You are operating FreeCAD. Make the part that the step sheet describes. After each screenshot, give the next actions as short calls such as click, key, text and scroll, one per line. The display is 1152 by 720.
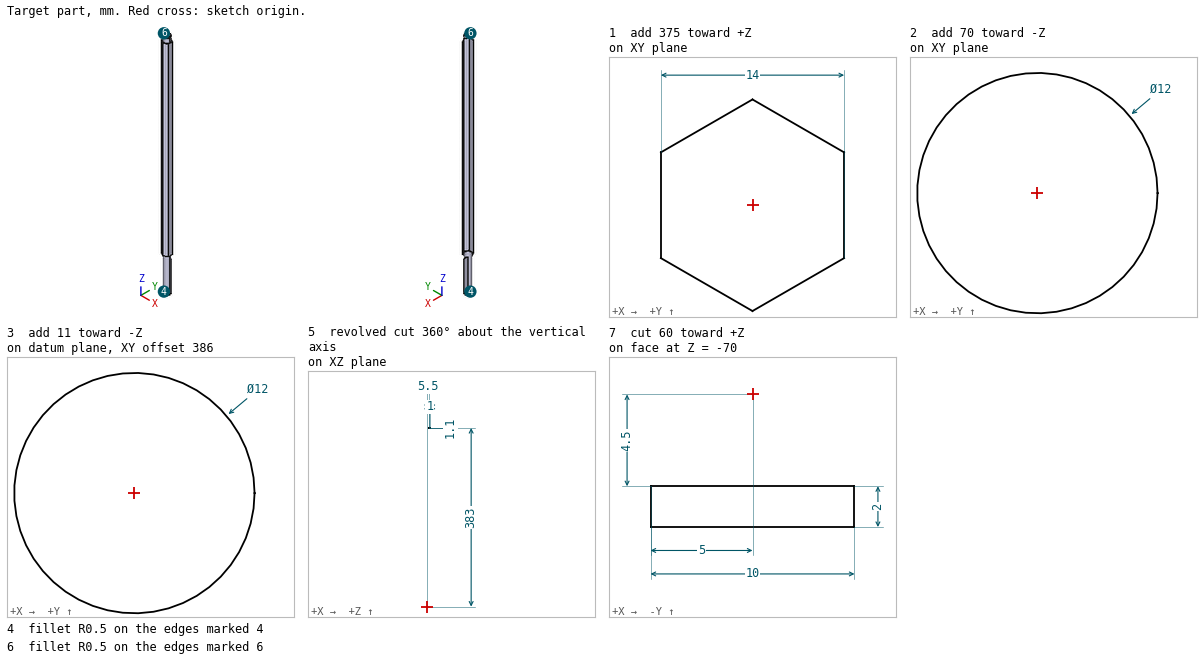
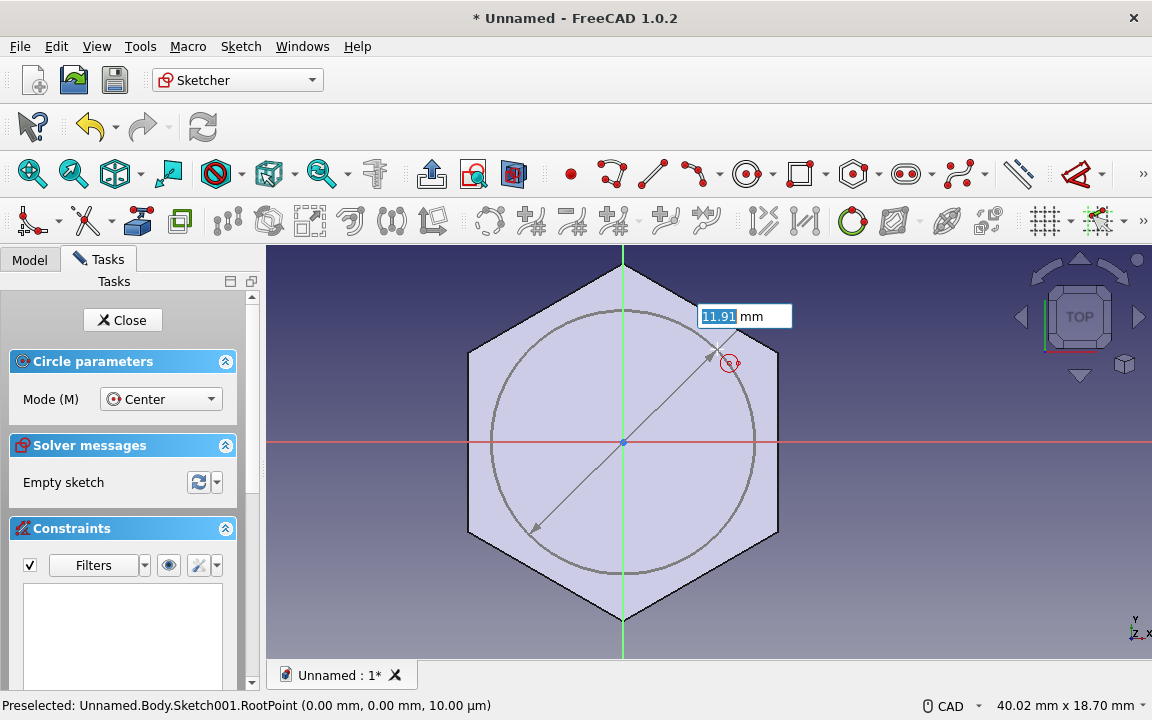
text(12)
key(Return)
key(Escape)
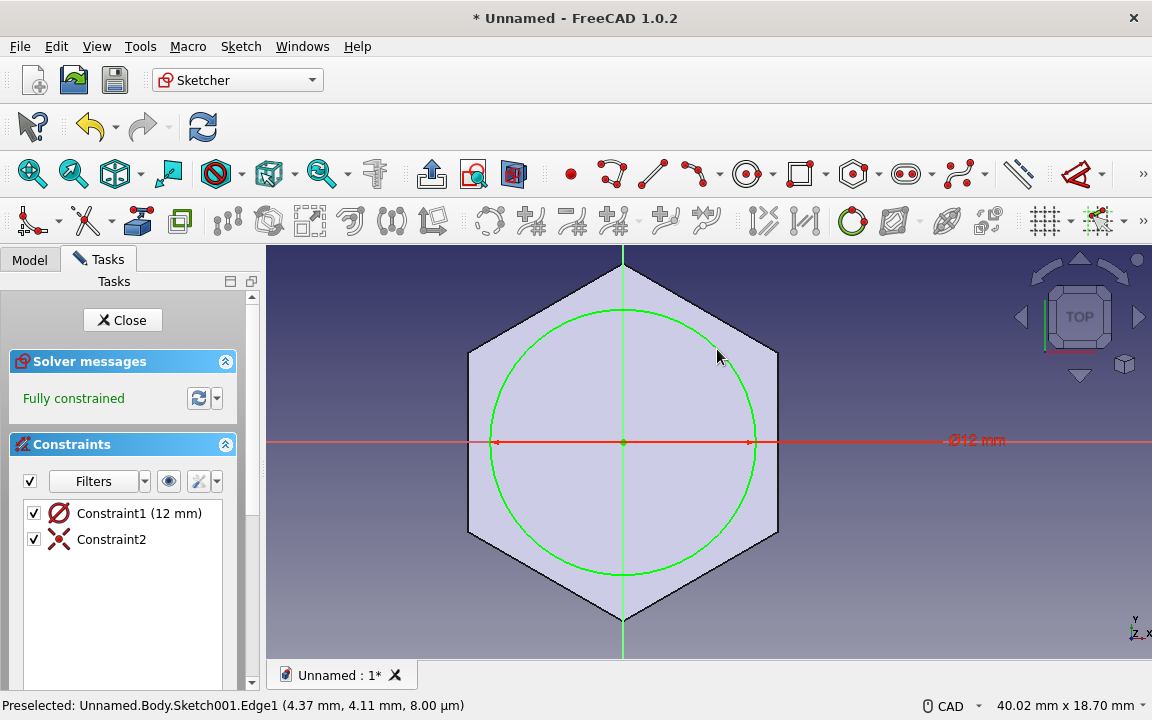
click(123, 320)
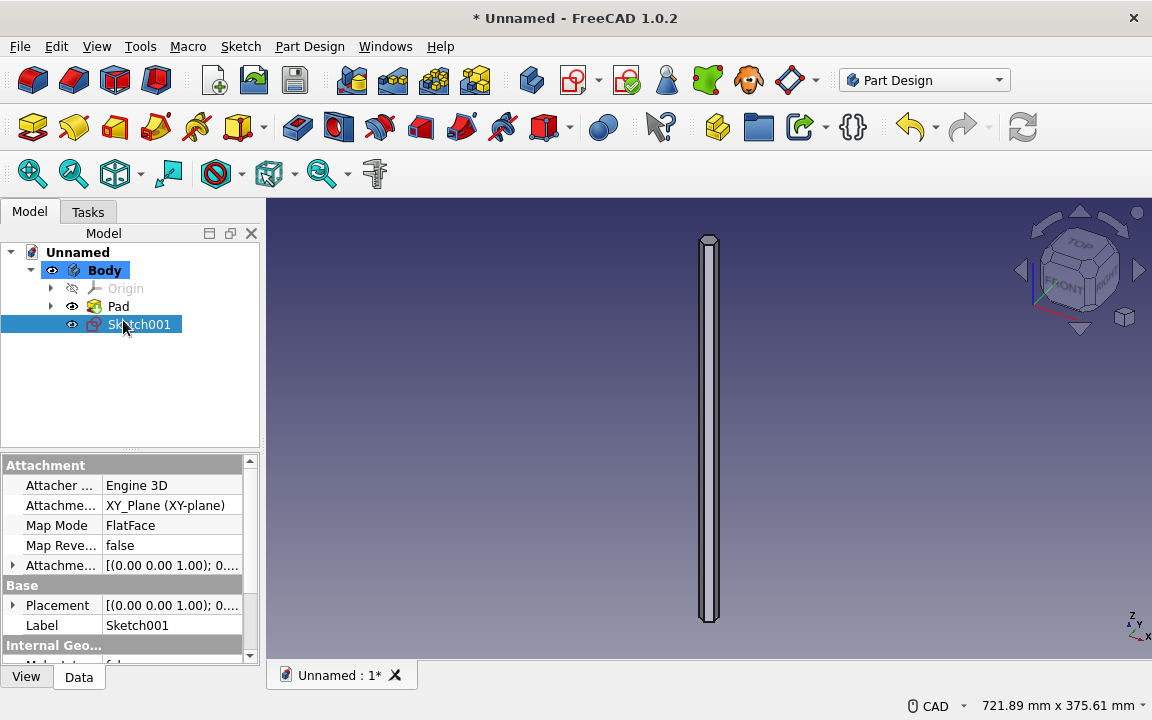
click(33, 128)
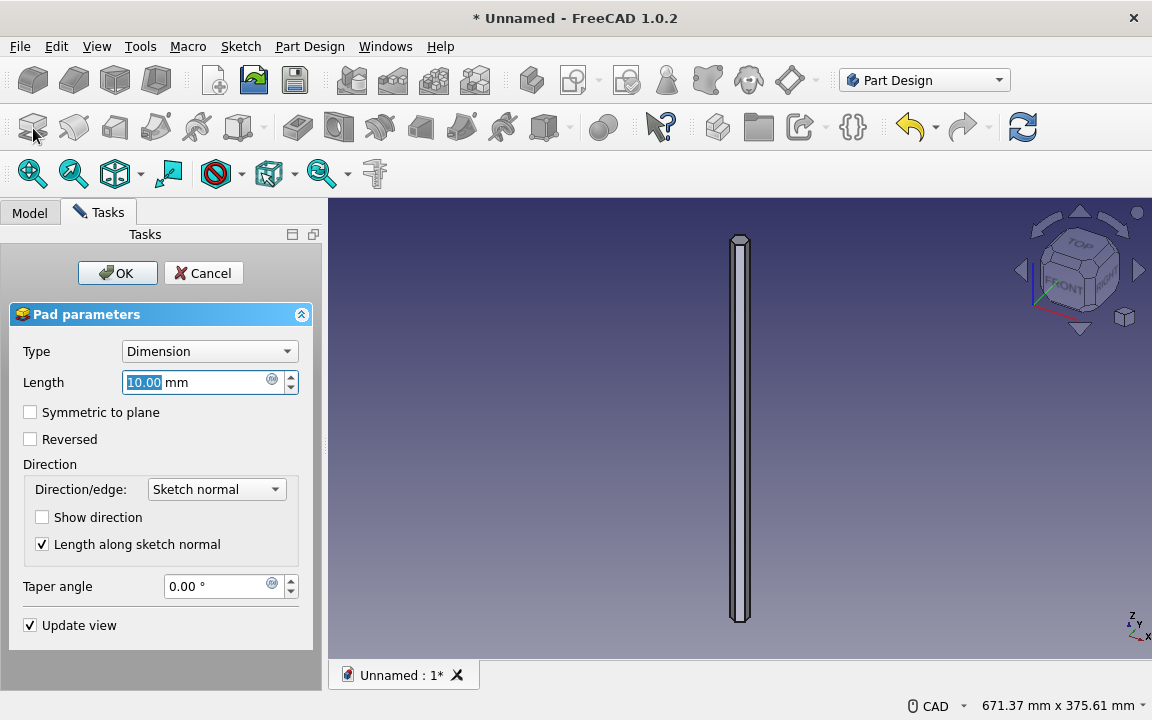
text(70)
key(Tab)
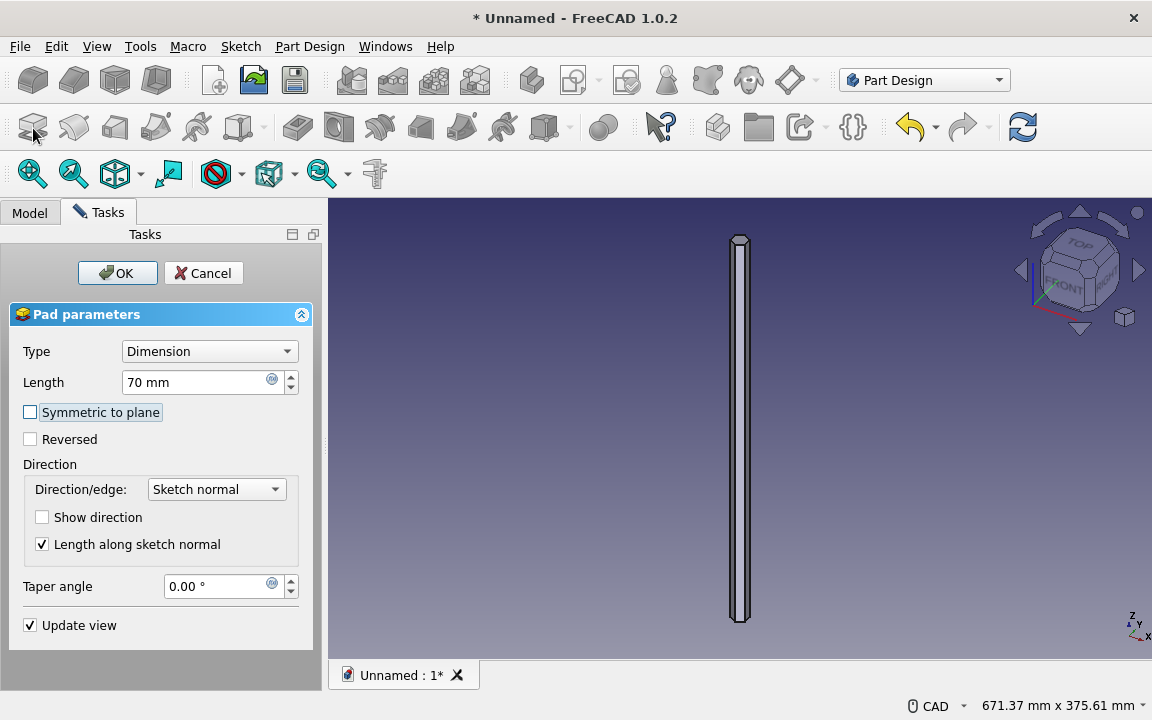
click(31, 439)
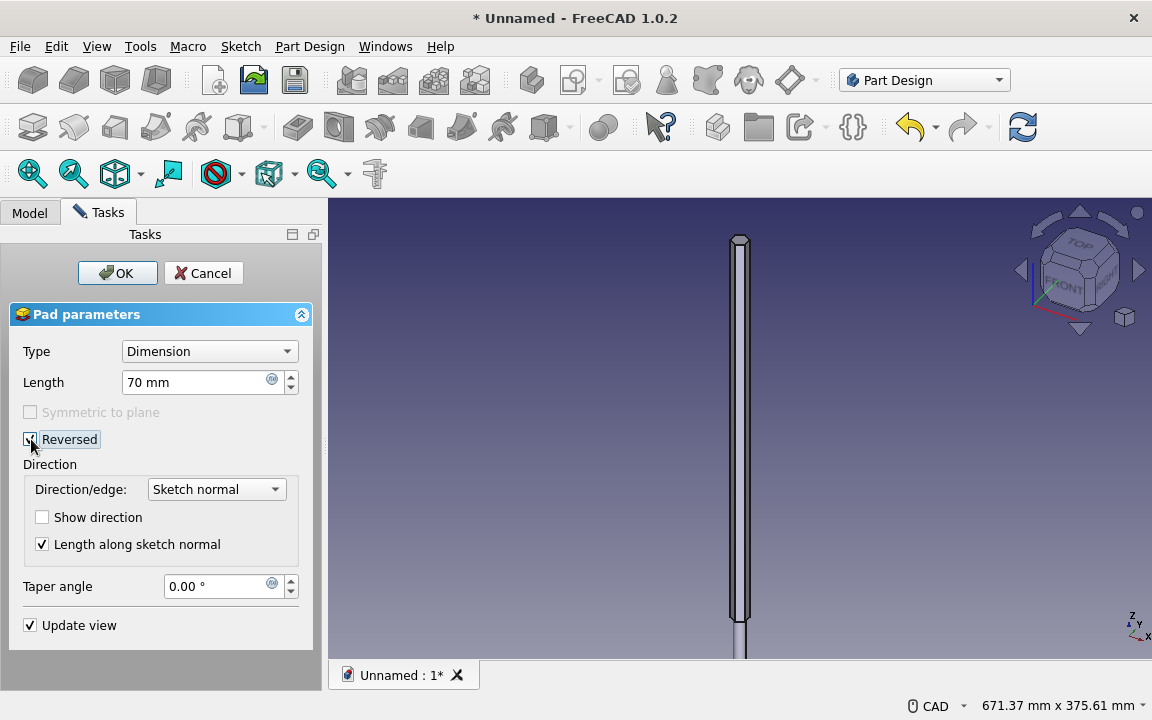
click(118, 273)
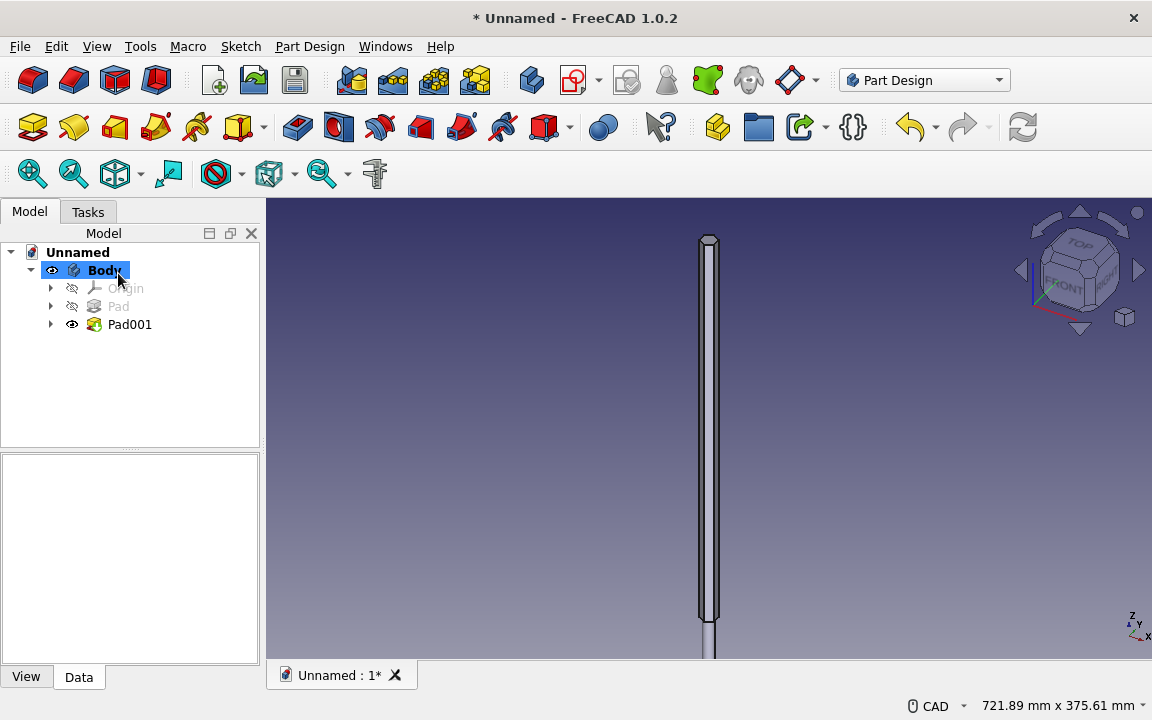
click(33, 174)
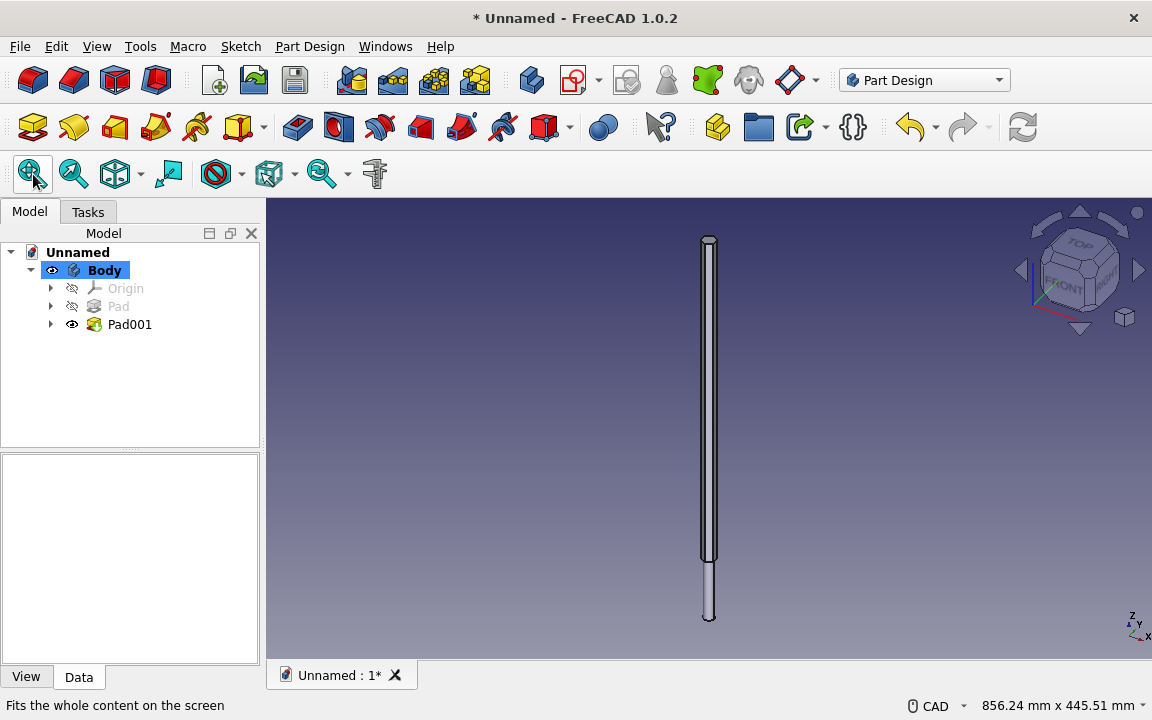
click(51, 288)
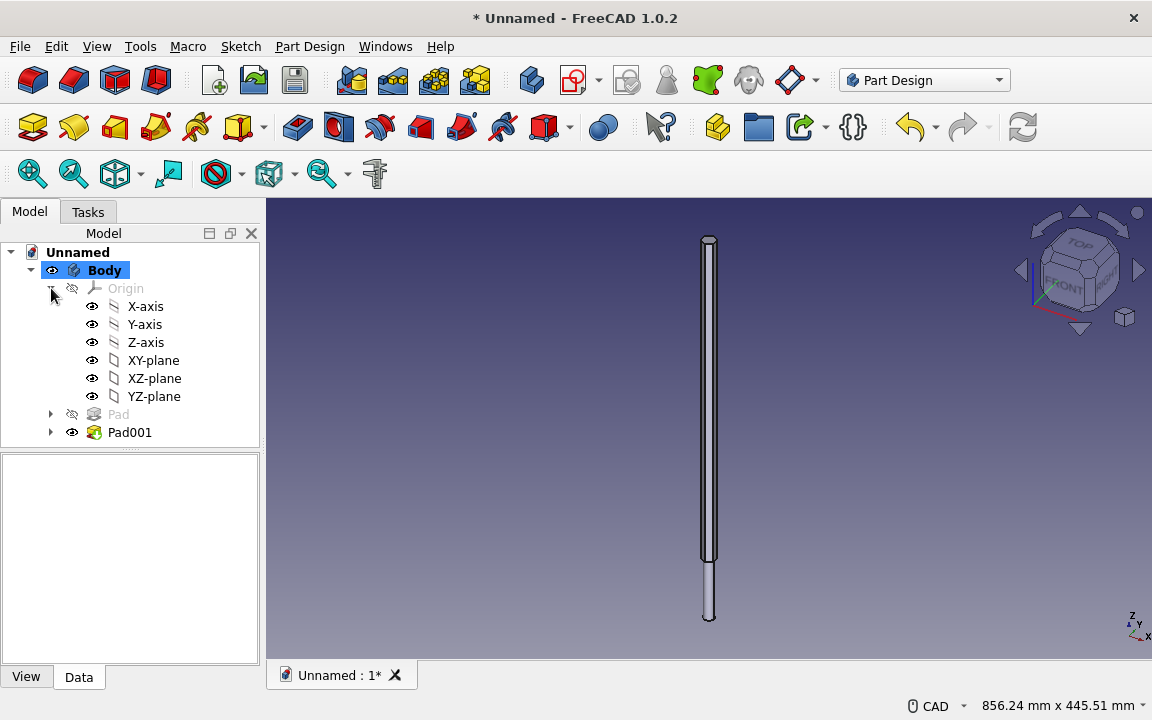
click(137, 360)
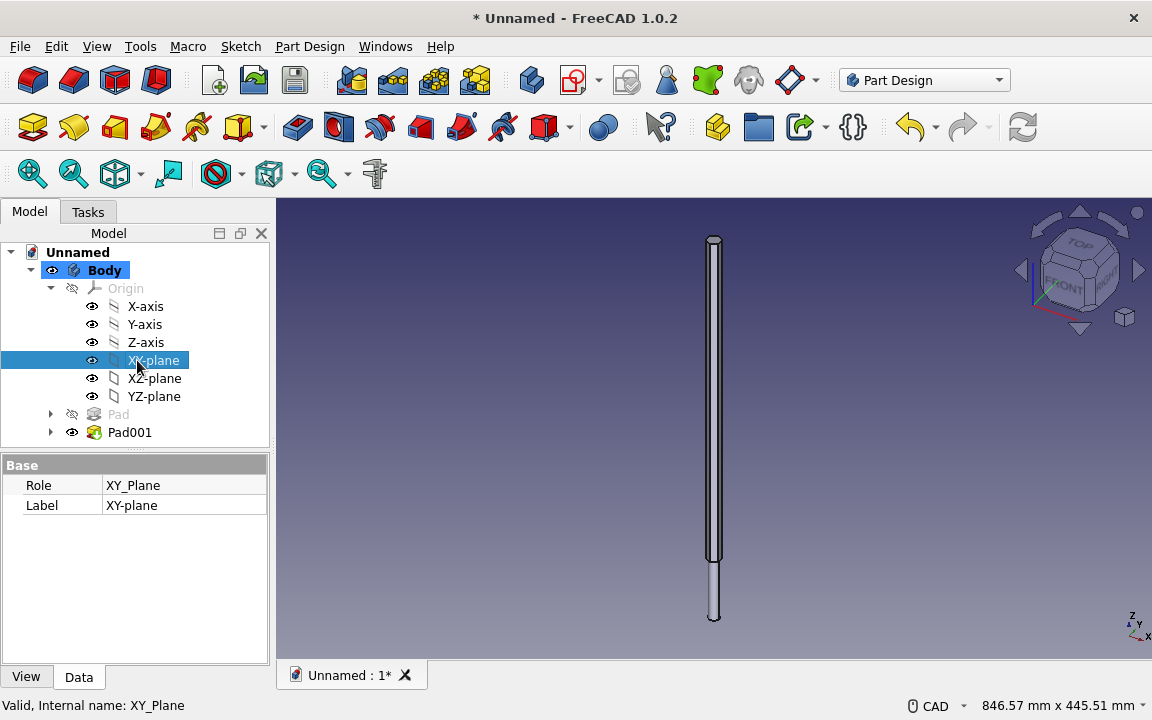
click(790, 80)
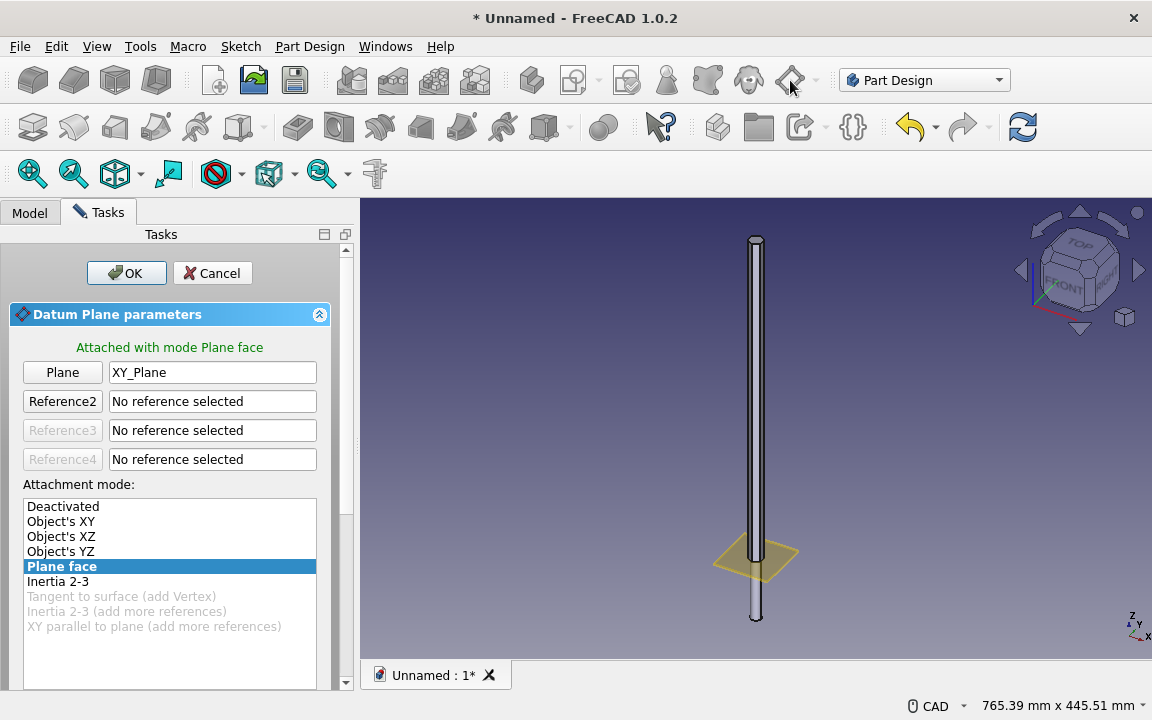
scroll(346, 467, down, 4)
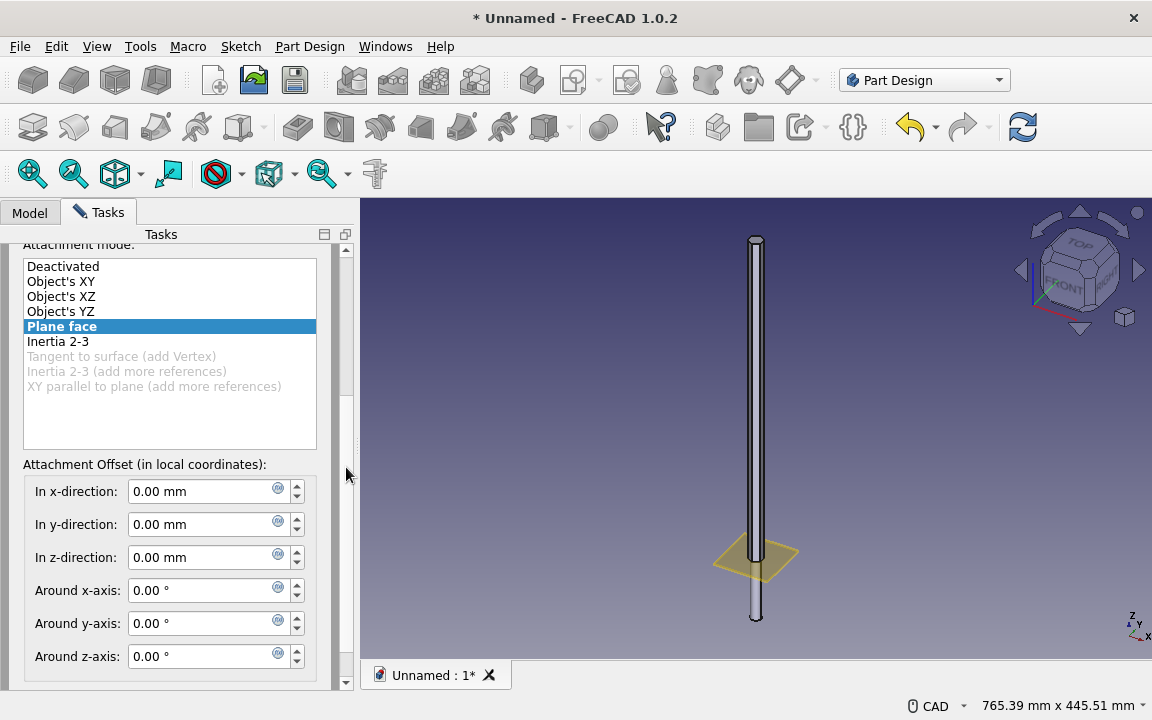
triple_click(210, 558)